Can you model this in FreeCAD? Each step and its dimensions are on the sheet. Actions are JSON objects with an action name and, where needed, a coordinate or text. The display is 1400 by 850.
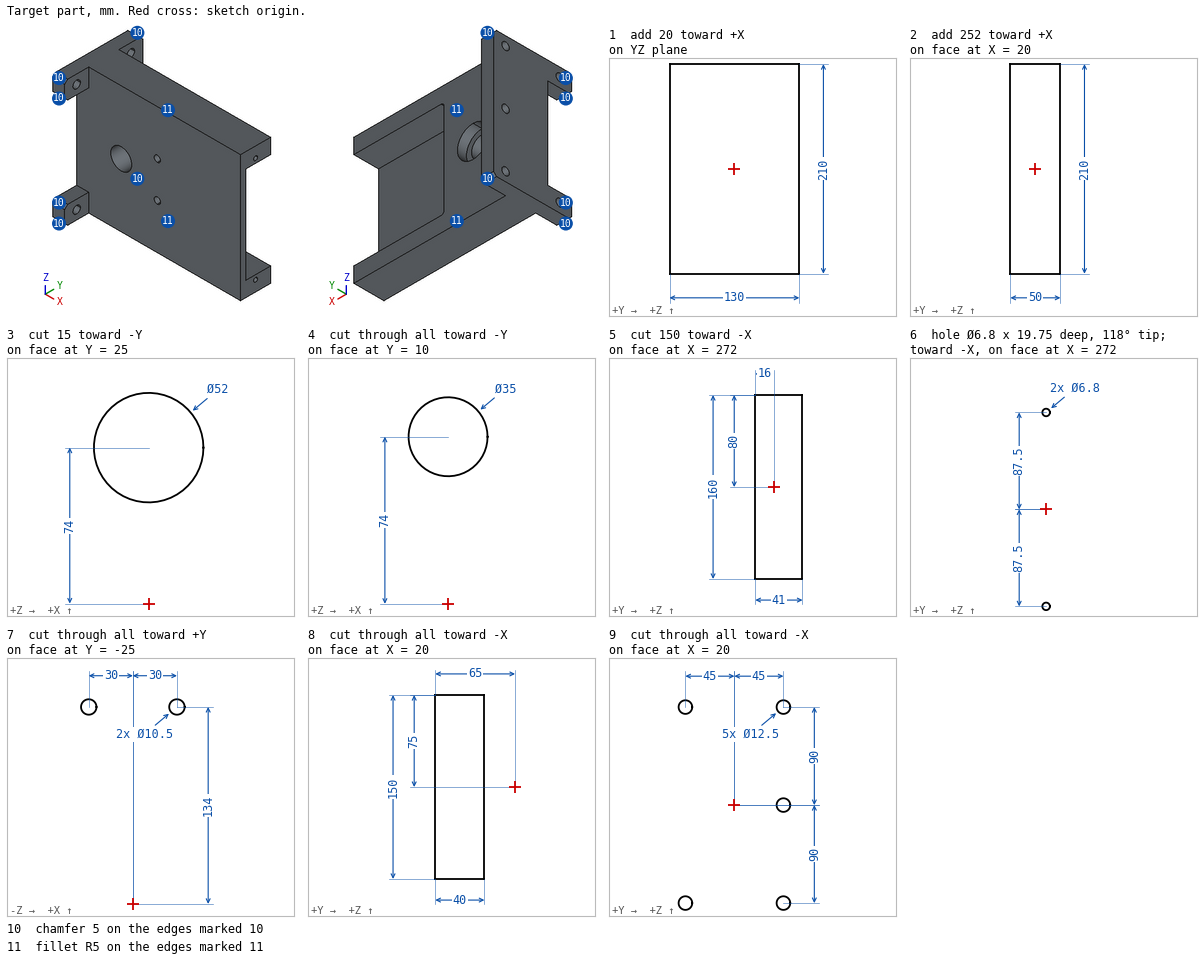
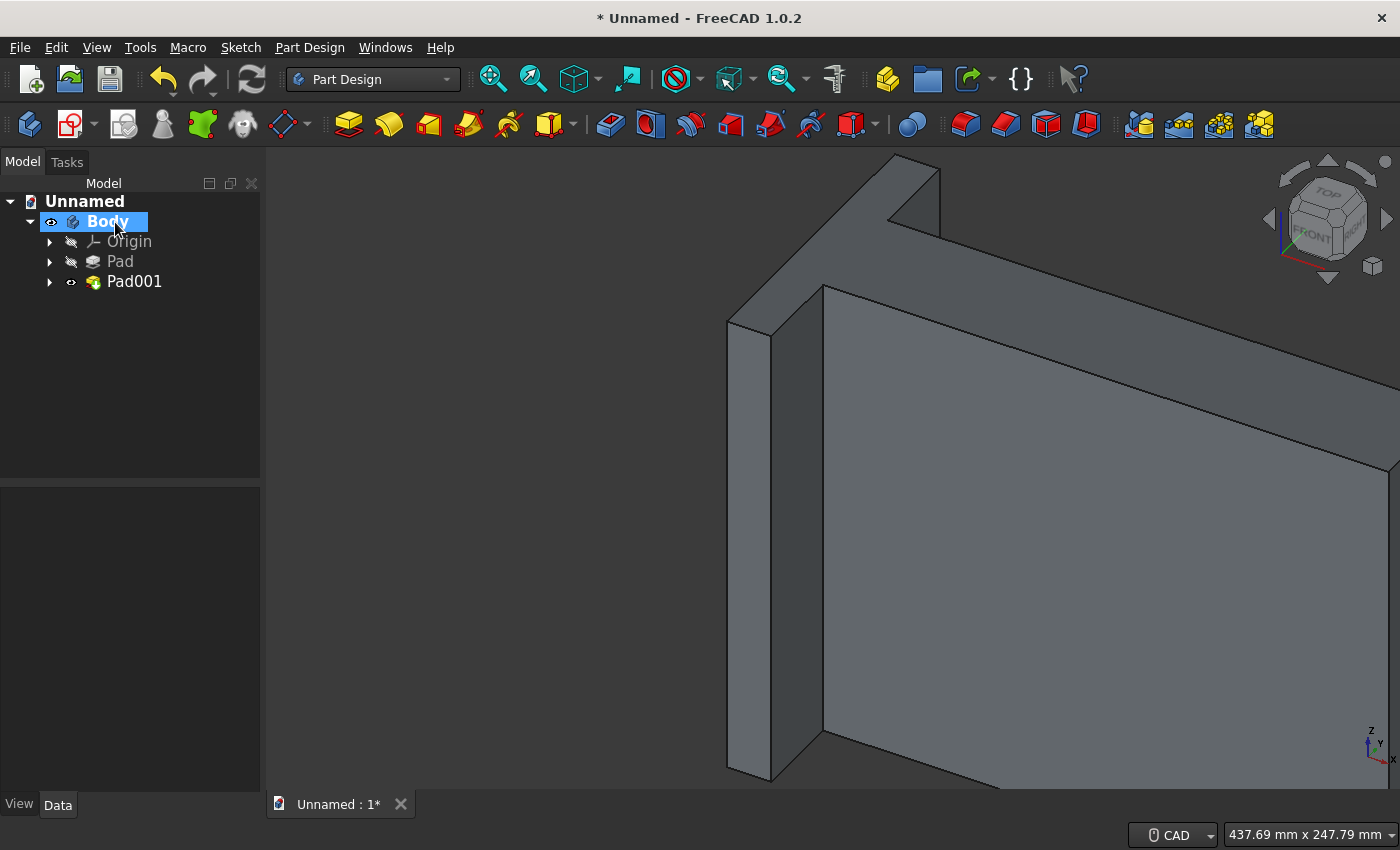
{"action": "left_click", "coordinate": [494, 80]}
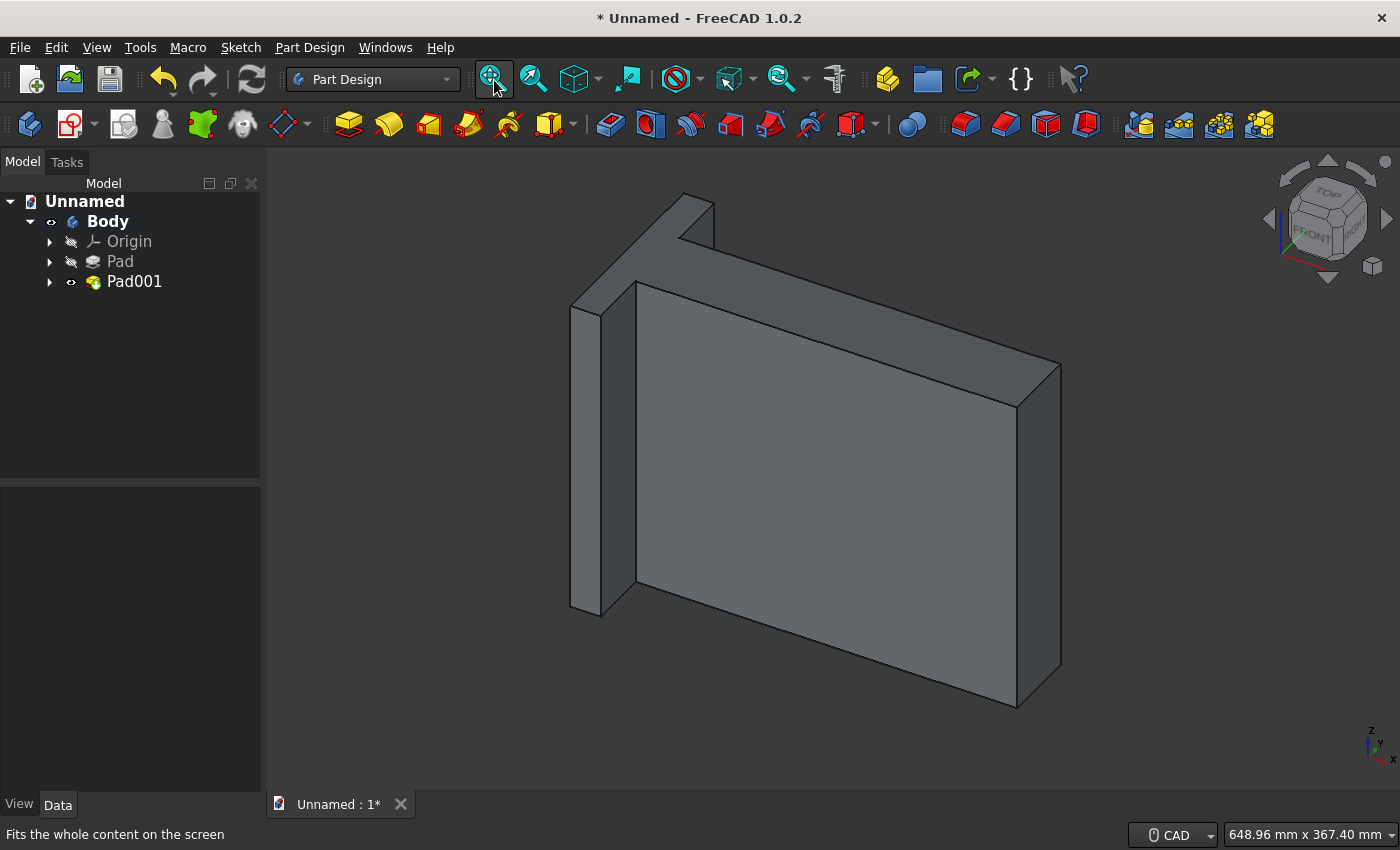
{"action": "key", "text": "4"}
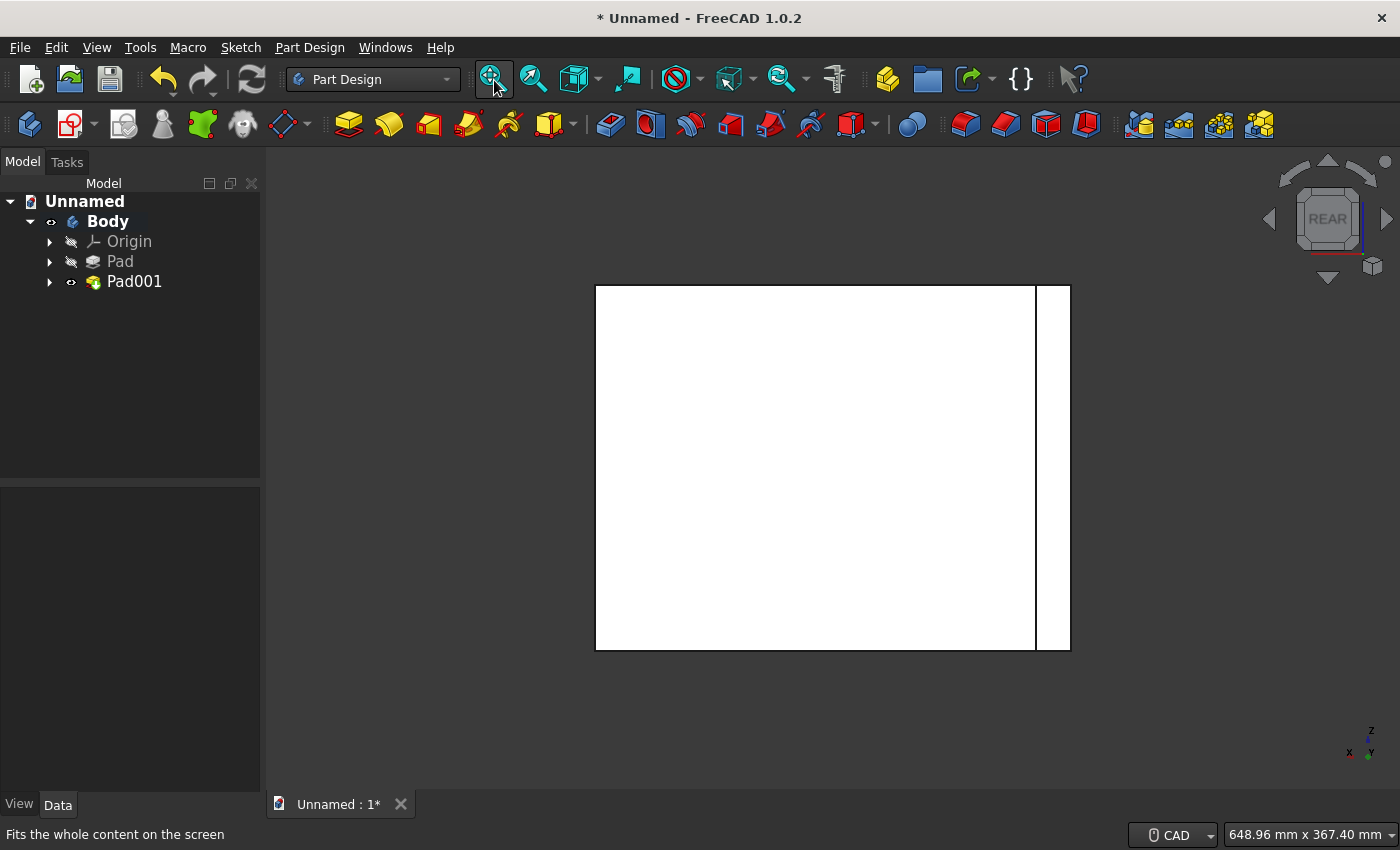
{"action": "left_click", "coordinate": [816, 467]}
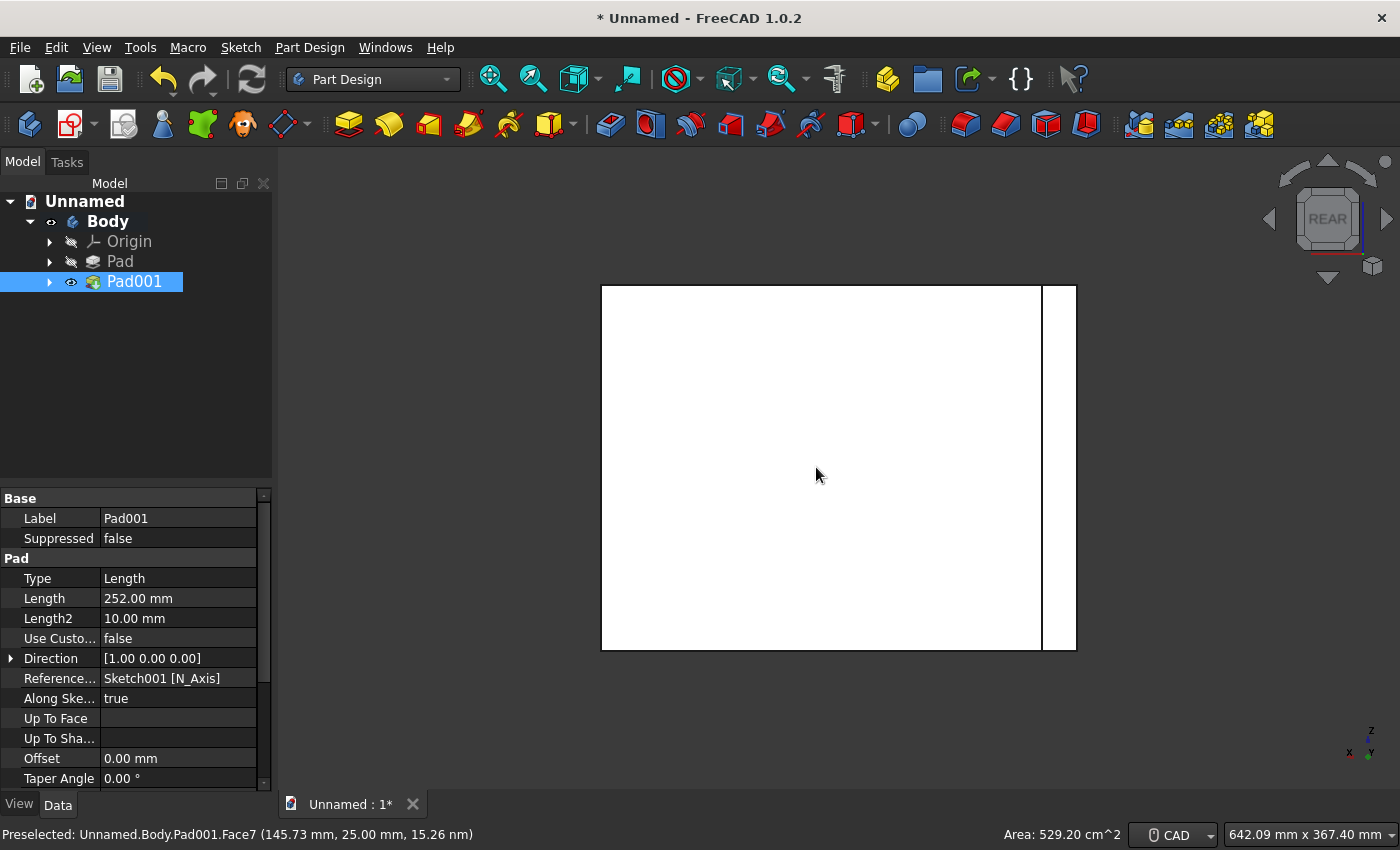
{"action": "left_click", "coordinate": [70, 124]}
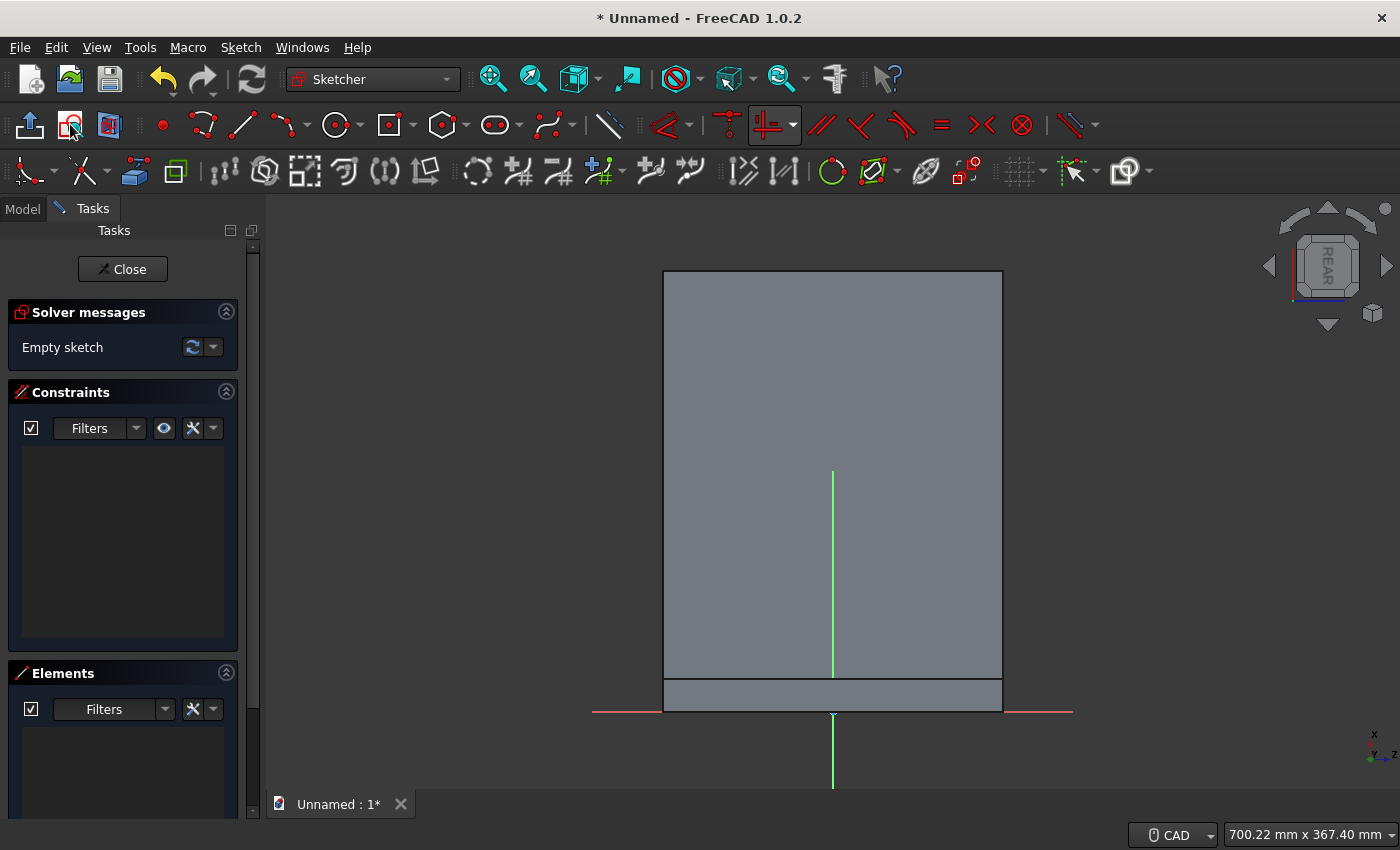
{"action": "left_click", "coordinate": [110, 126]}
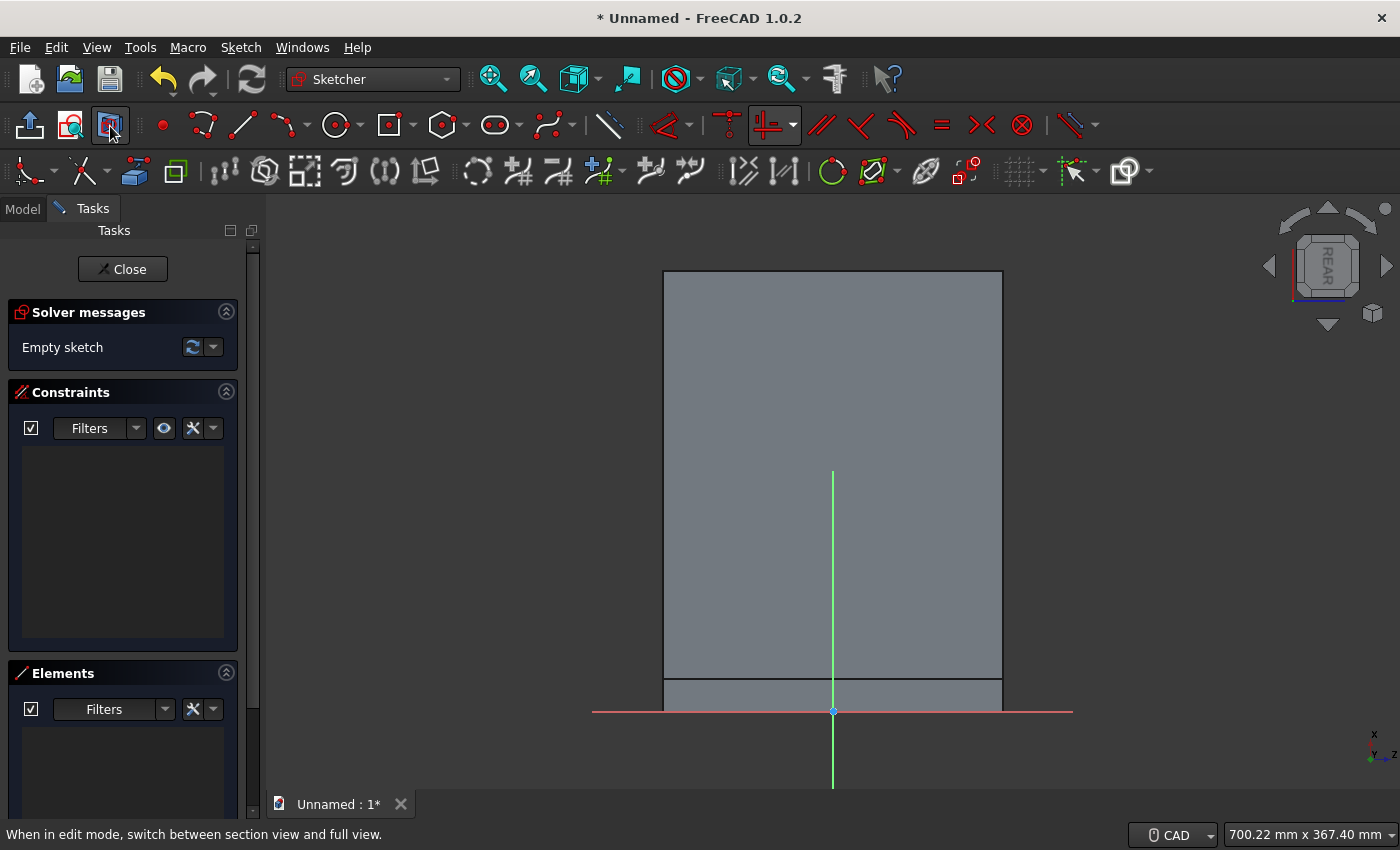
{"action": "scroll", "coordinate": [889, 744], "scroll_direction": "up", "scroll_amount": 4}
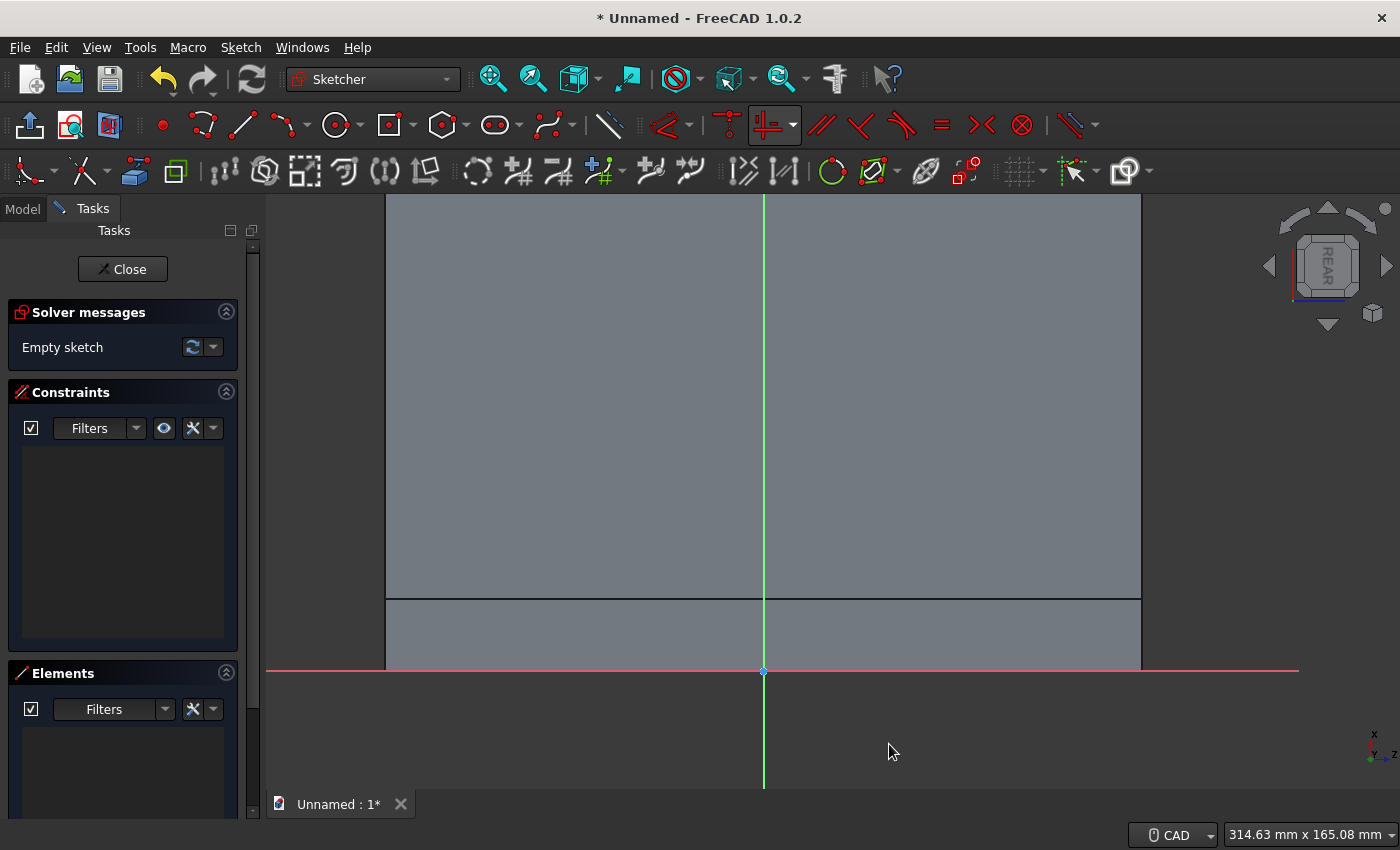
{"action": "left_click", "coordinate": [336, 126]}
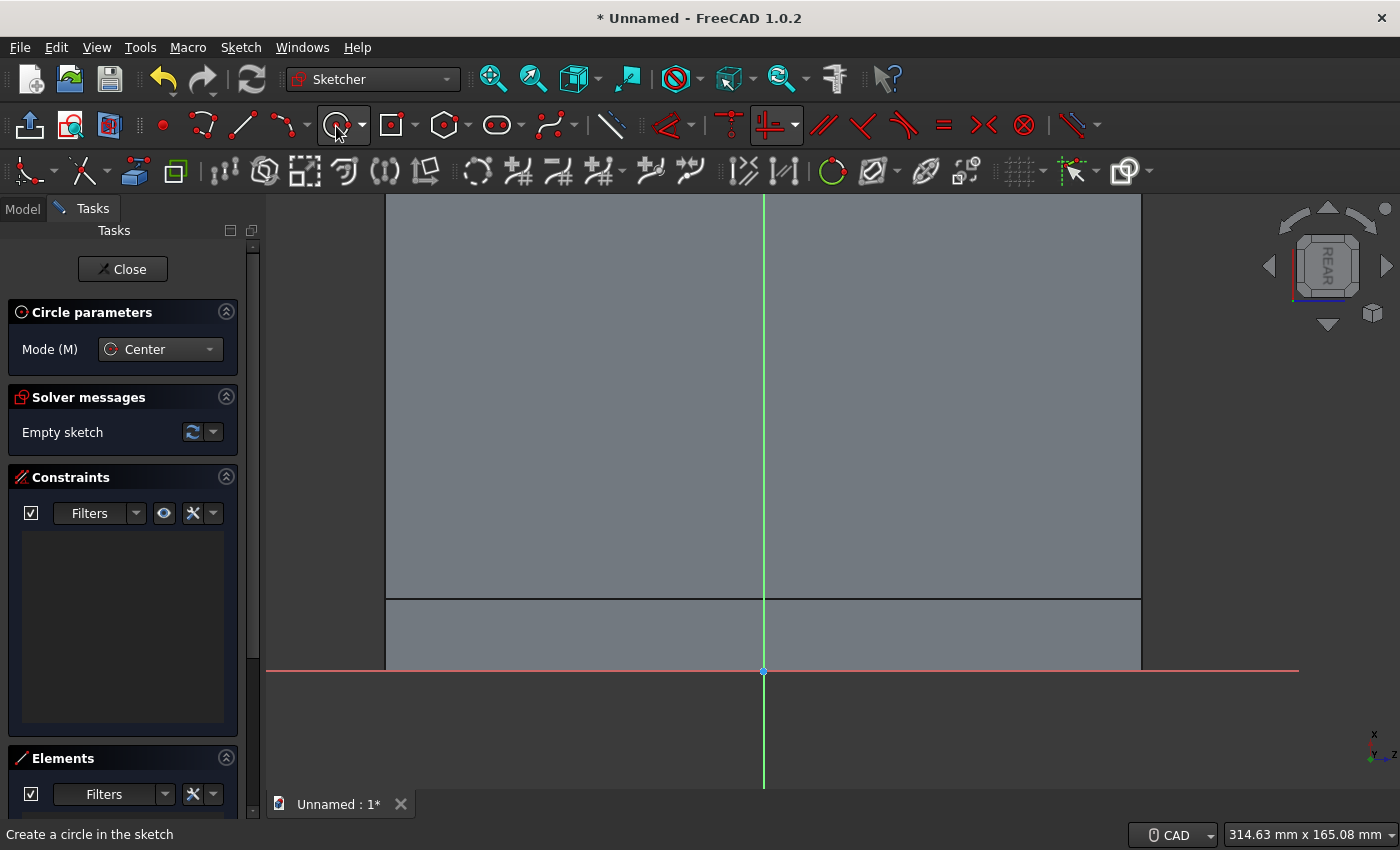
{"action": "left_click", "coordinate": [764, 404]}
{"action": "left_click", "coordinate": [830, 338]}
{"action": "key", "text": "Escape"}